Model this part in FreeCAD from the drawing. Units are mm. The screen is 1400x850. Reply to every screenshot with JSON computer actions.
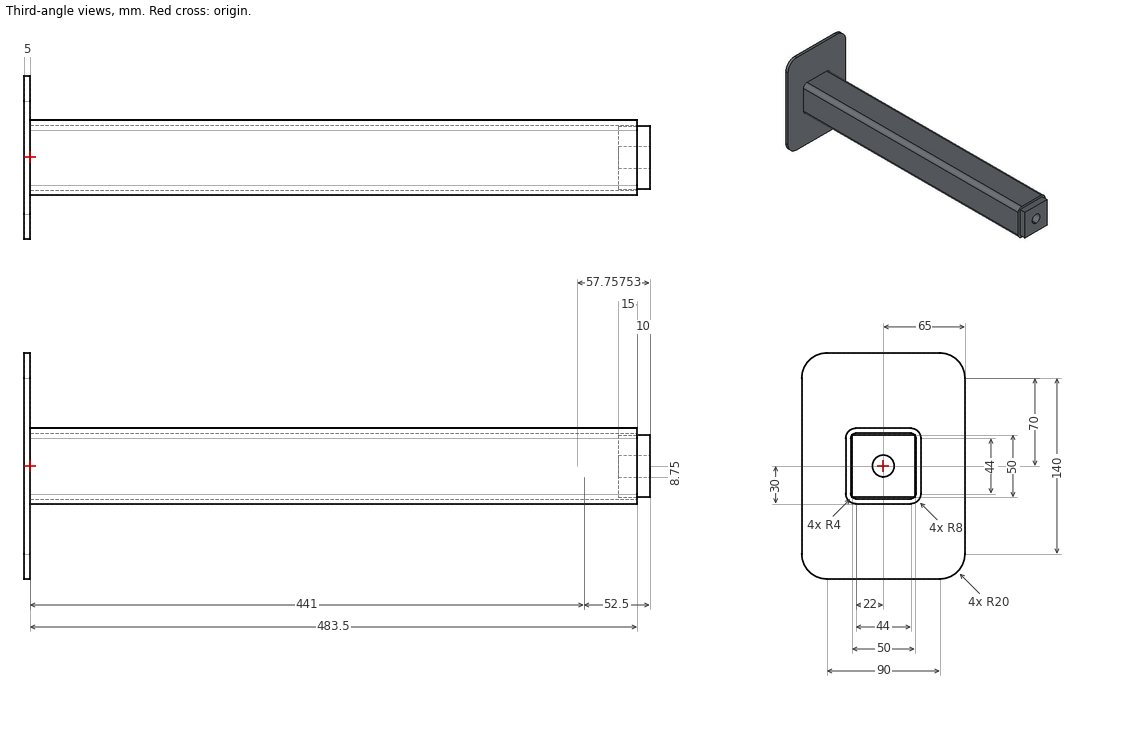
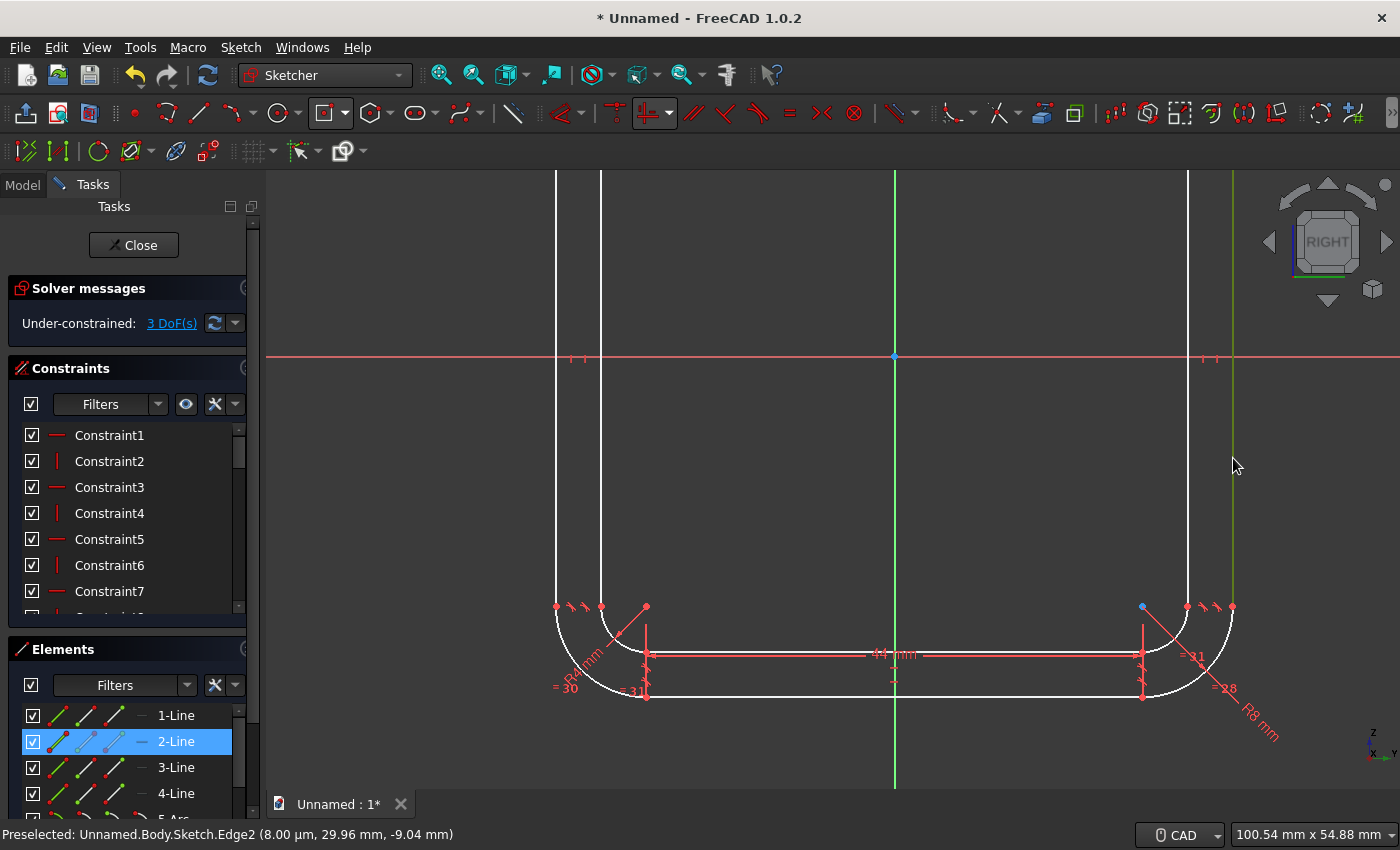
{"action": "key", "text": "i"}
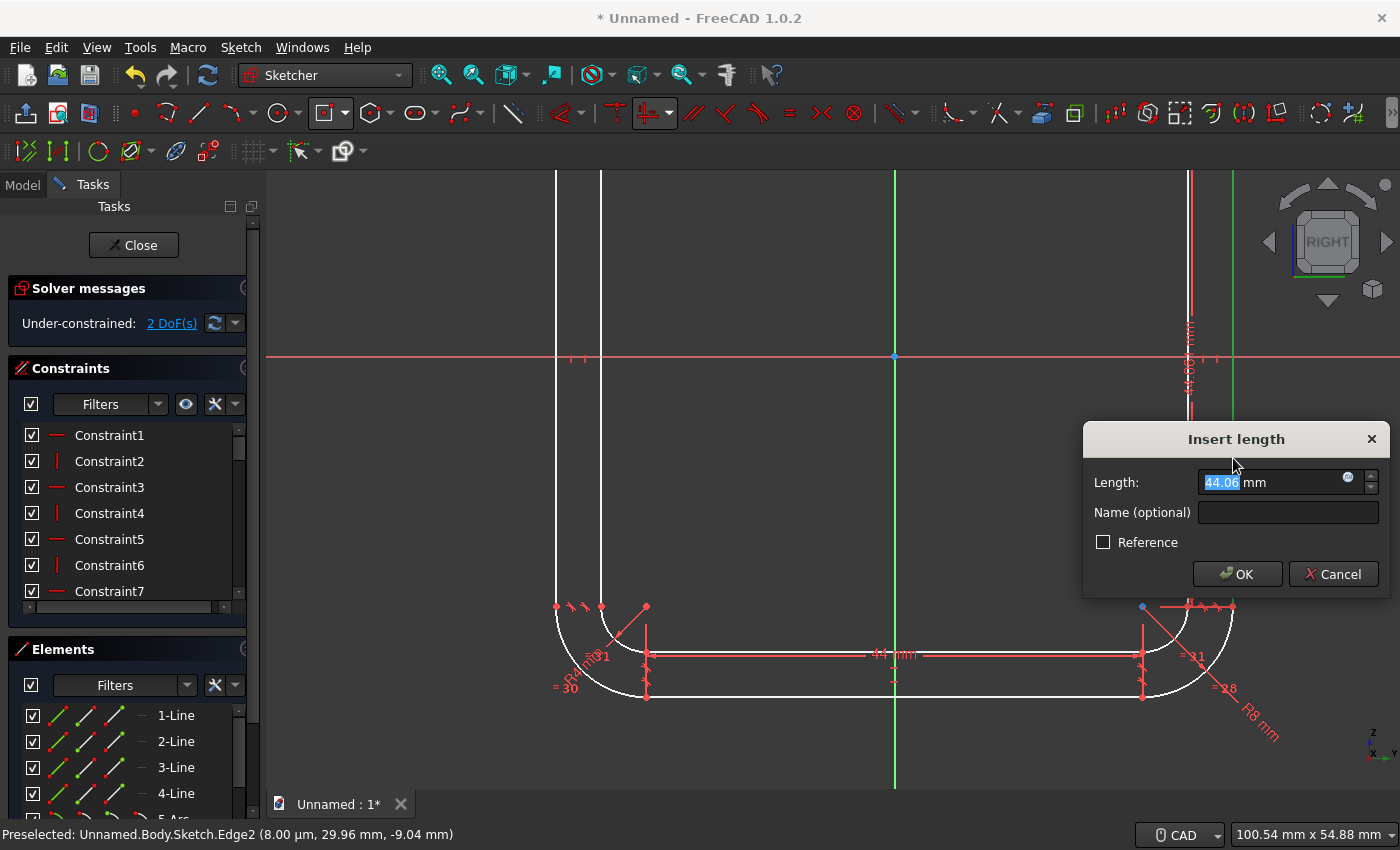
{"action": "type", "text": "44"}
{"action": "key", "text": "Return"}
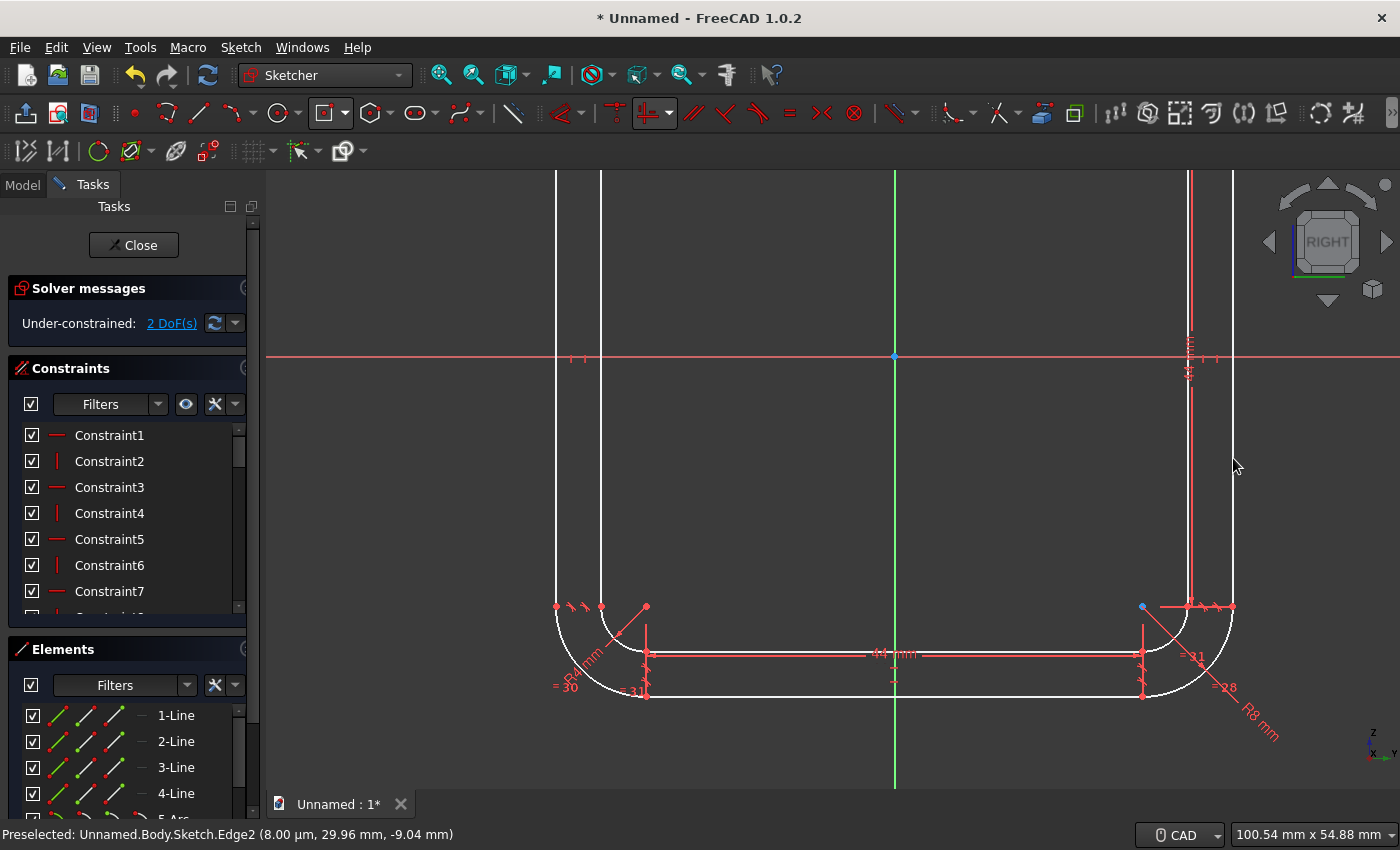
{"action": "left_click", "coordinate": [646, 697]}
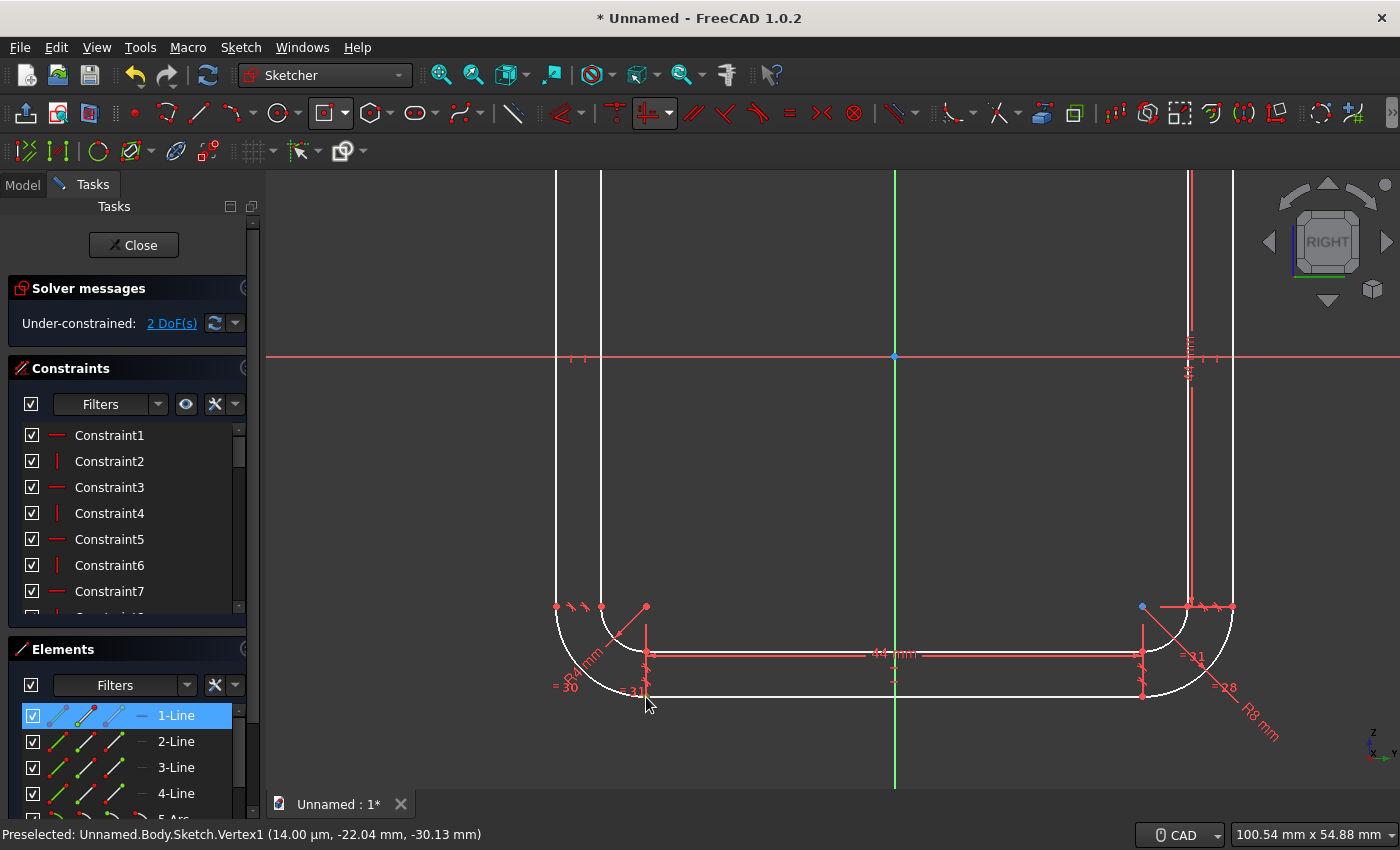
{"action": "key", "text": "l"}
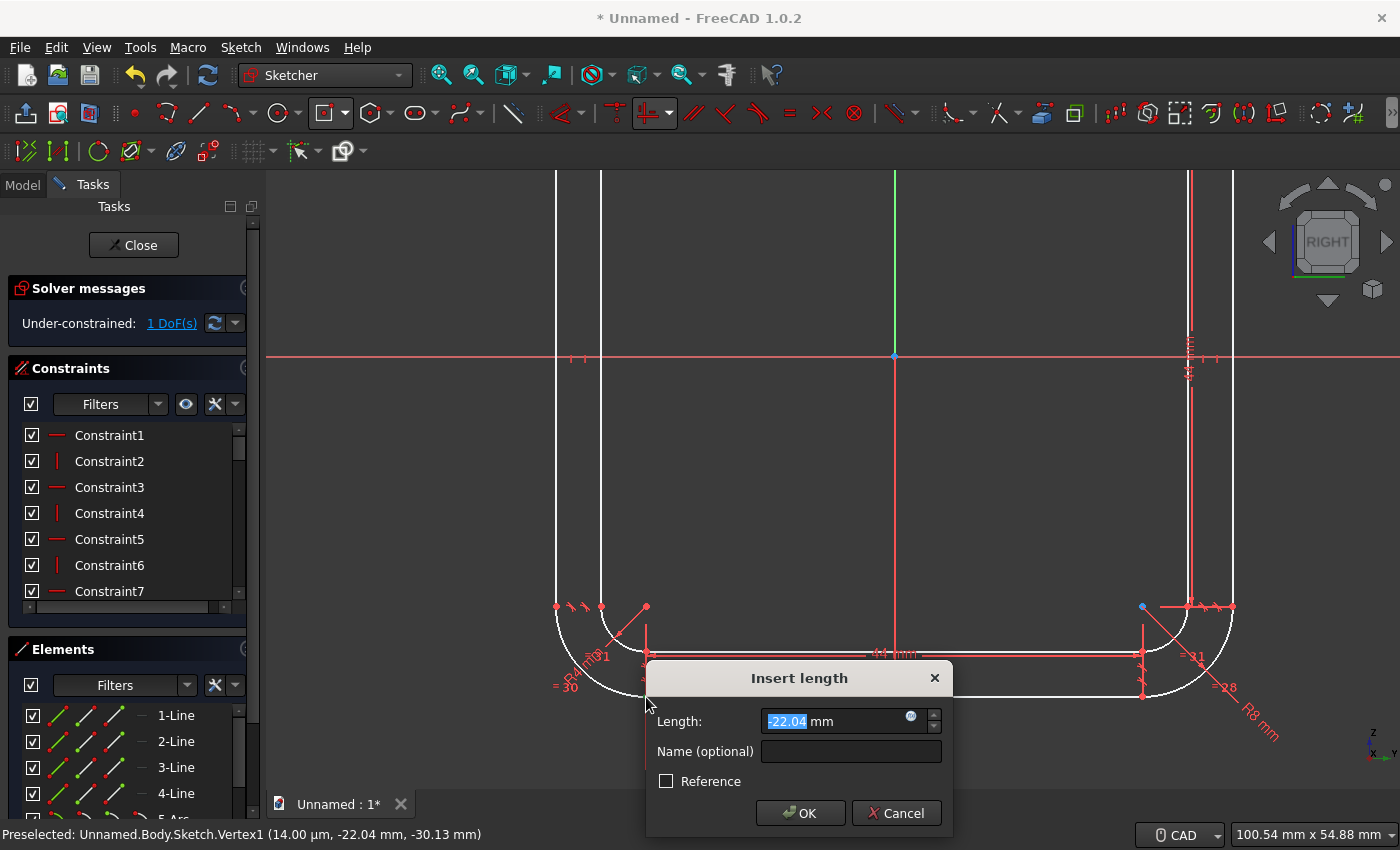
{"action": "type", "text": "-22"}
{"action": "key", "text": "Return"}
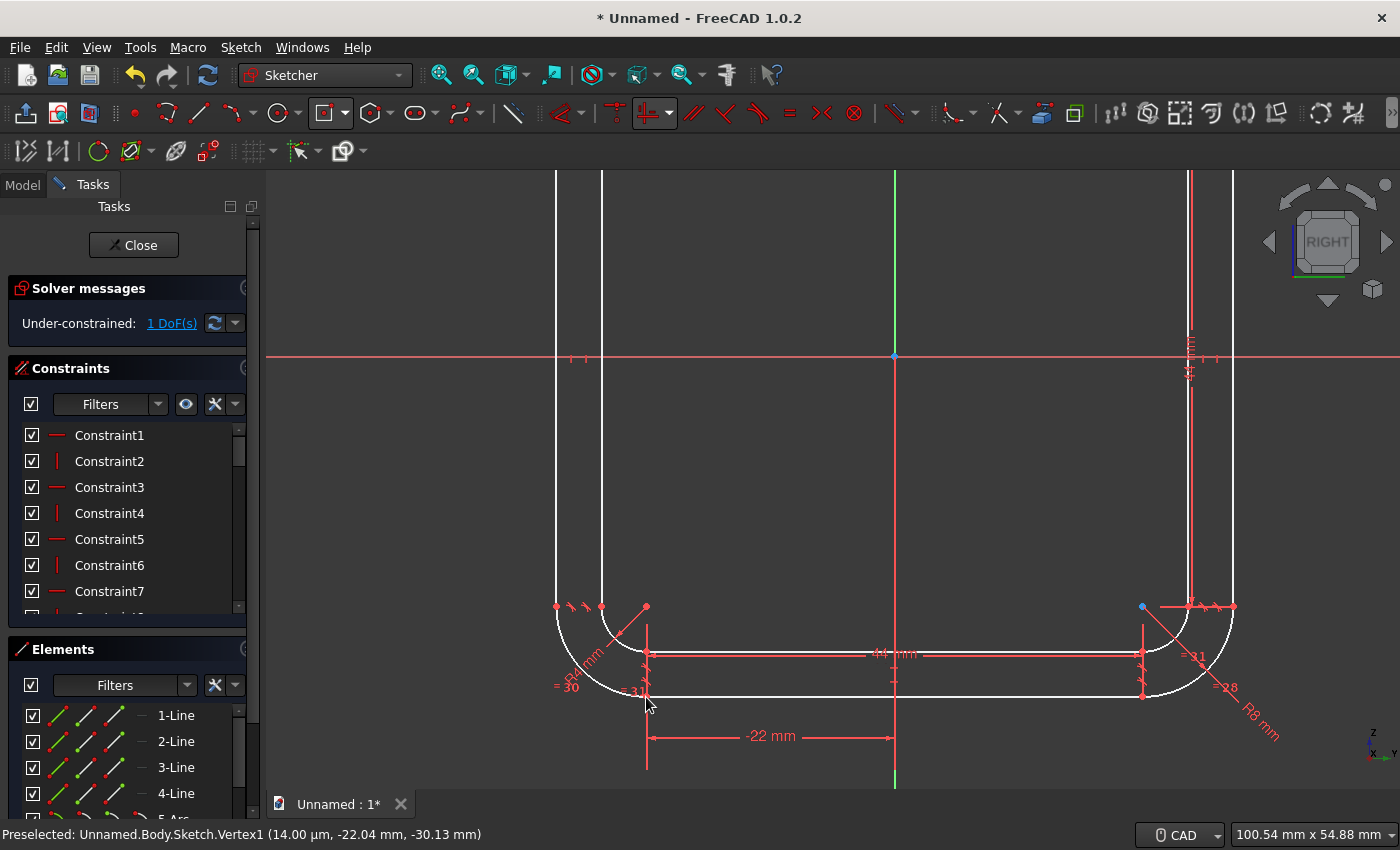
{"action": "left_click", "coordinate": [647, 697]}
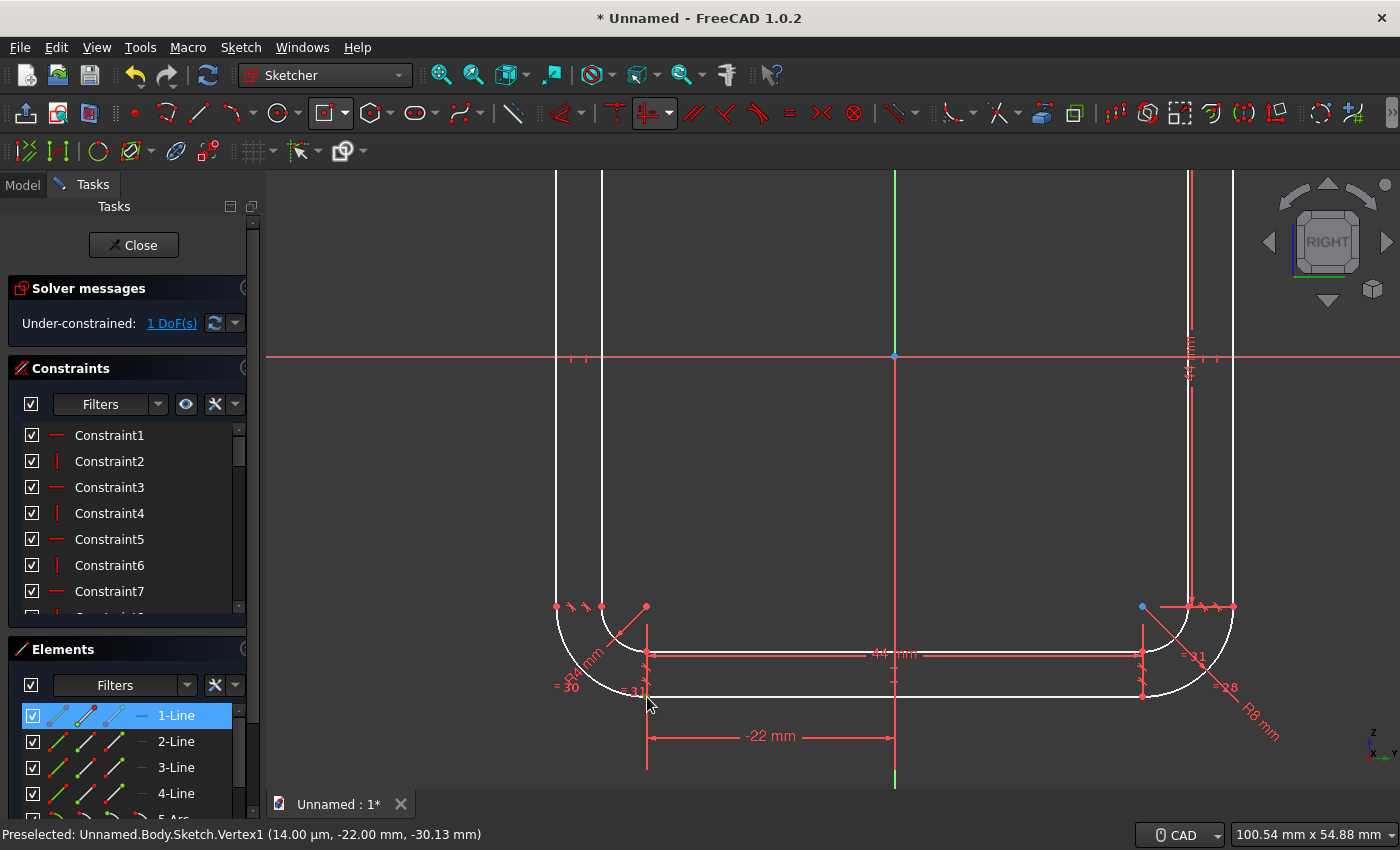
{"action": "left_click", "coordinate": [584, 114]}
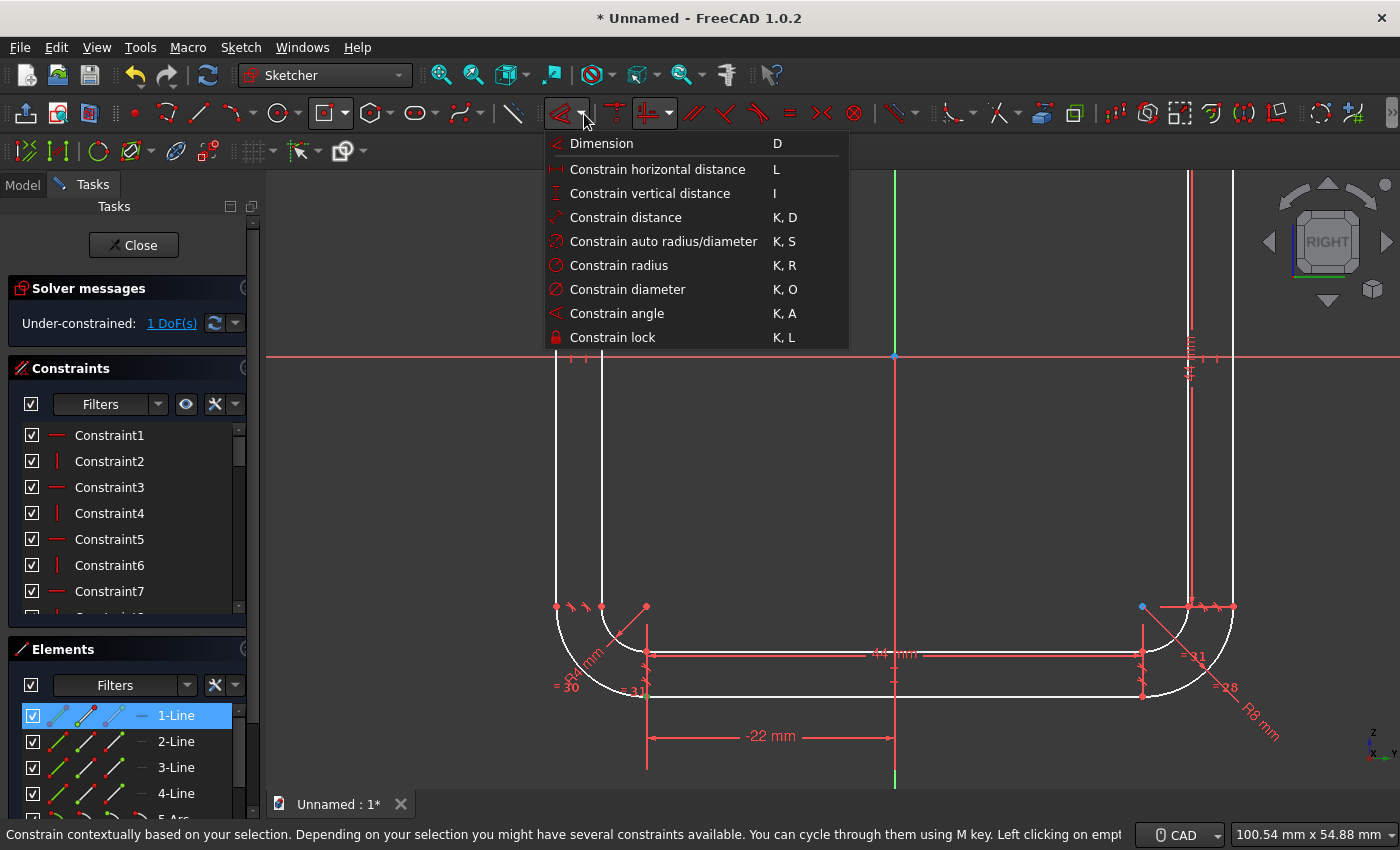
{"action": "left_click", "coordinate": [697, 193]}